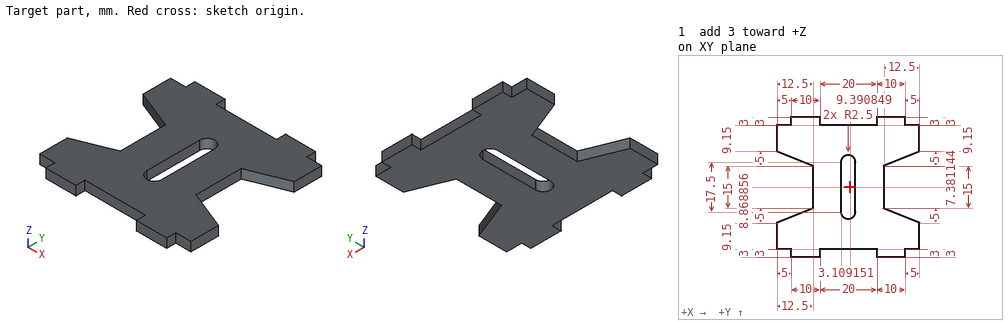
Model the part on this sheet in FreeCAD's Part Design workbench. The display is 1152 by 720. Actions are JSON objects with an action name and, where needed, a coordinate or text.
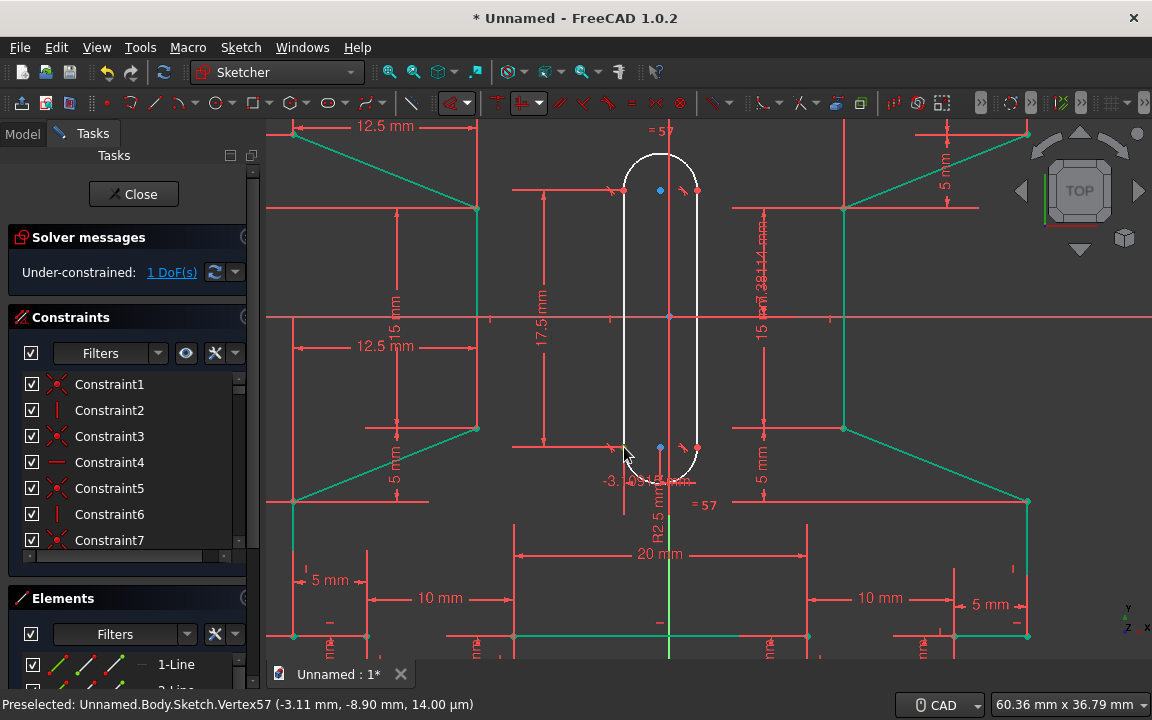
{"action": "key", "text": "i"}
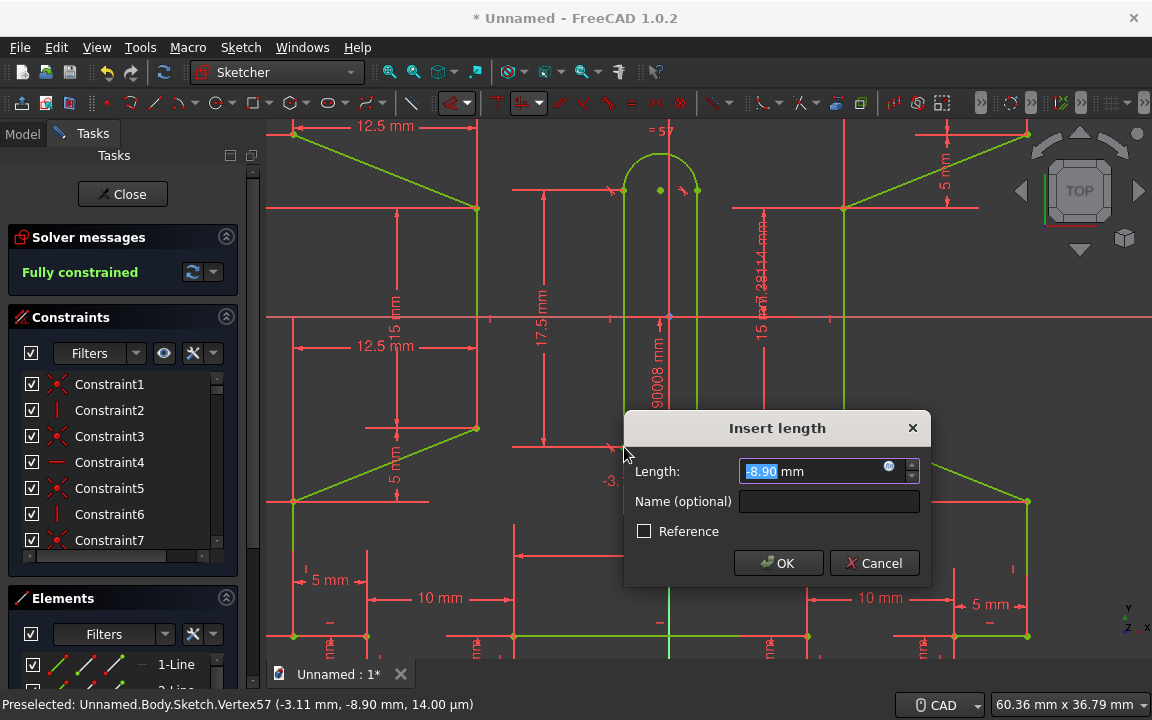
{"action": "type", "text": "-8.868856"}
{"action": "key", "text": "Return"}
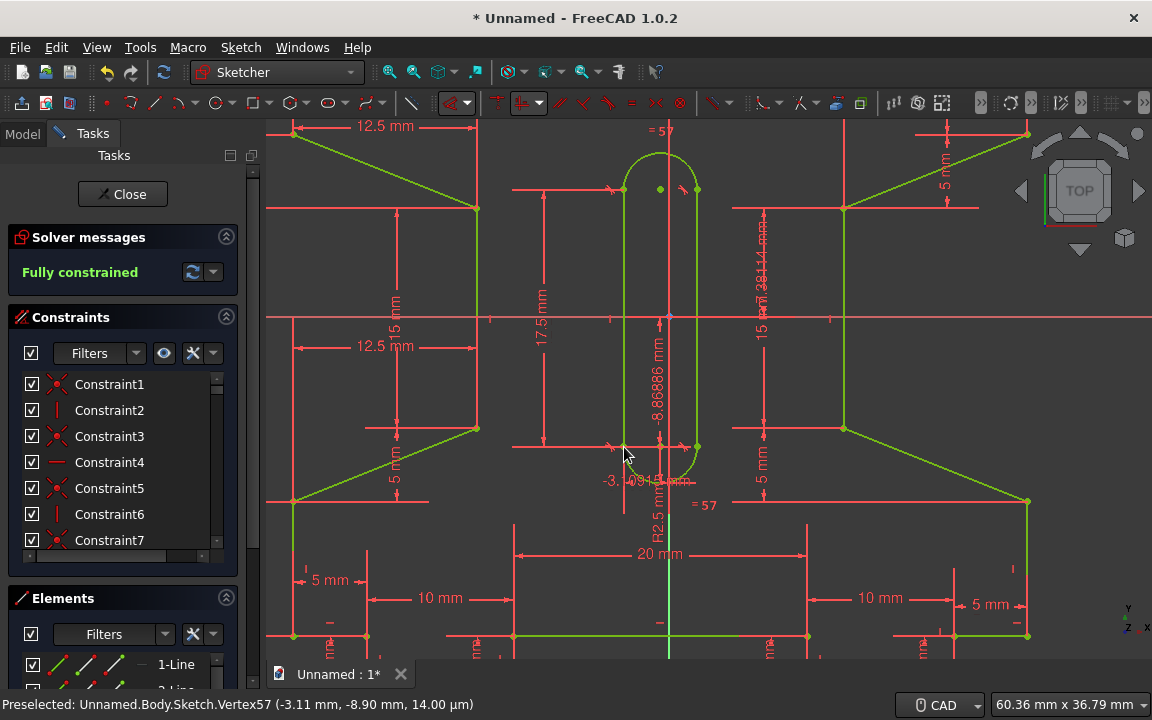
{"action": "left_click", "coordinate": [123, 194]}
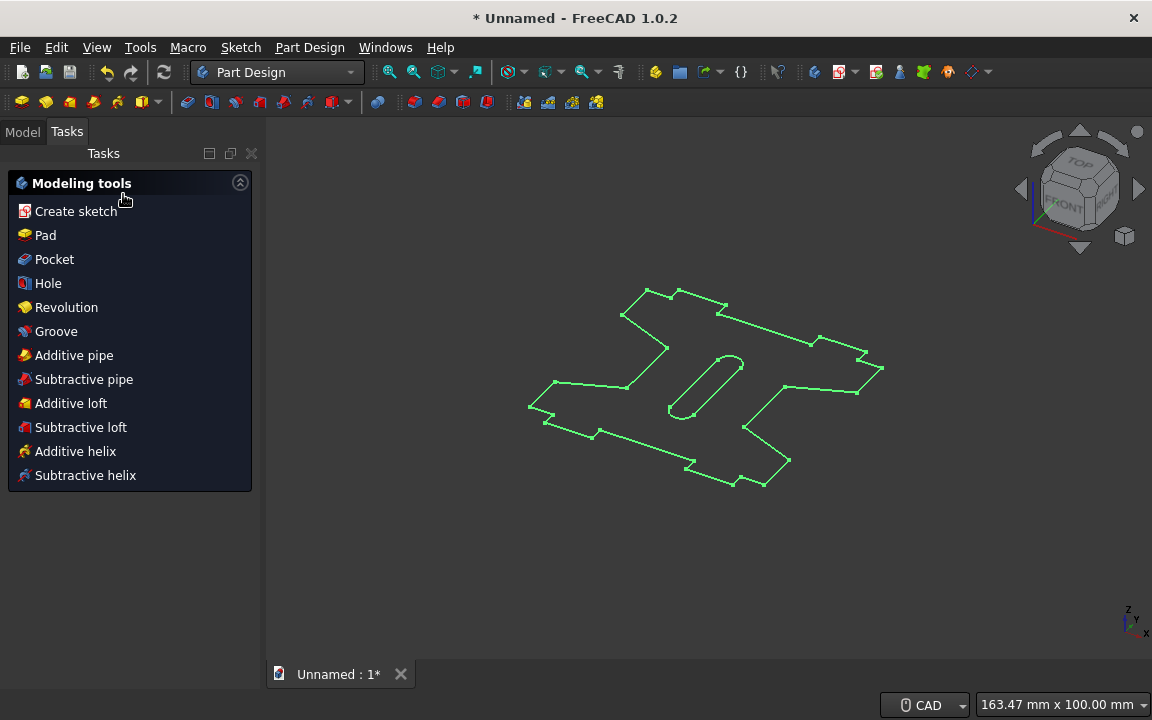
{"action": "left_click", "coordinate": [22, 102]}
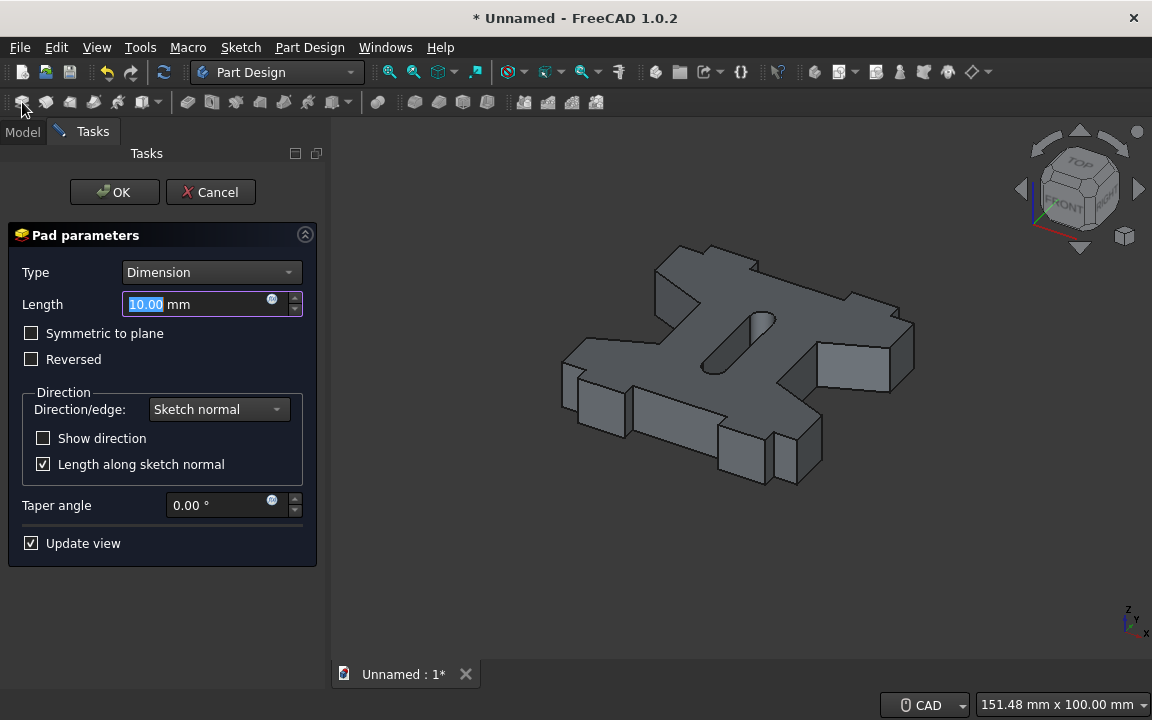
{"action": "type", "text": "3"}
{"action": "key", "text": "Tab"}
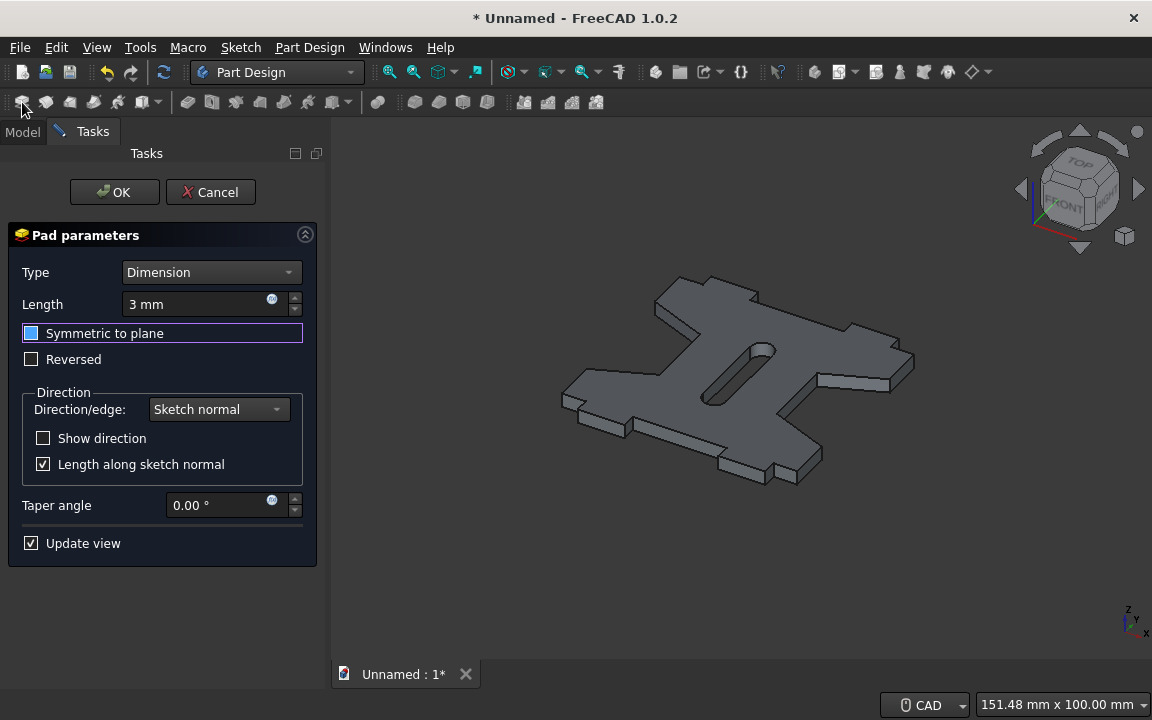
{"action": "left_click", "coordinate": [115, 192]}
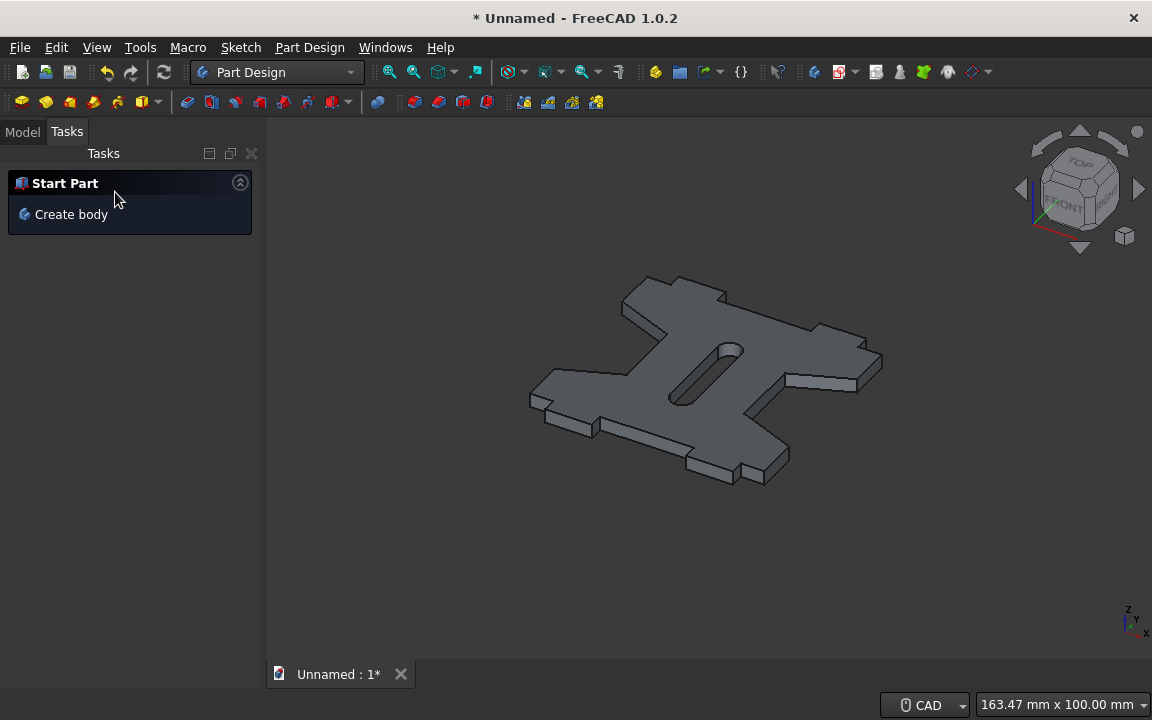
{"action": "key", "text": "0"}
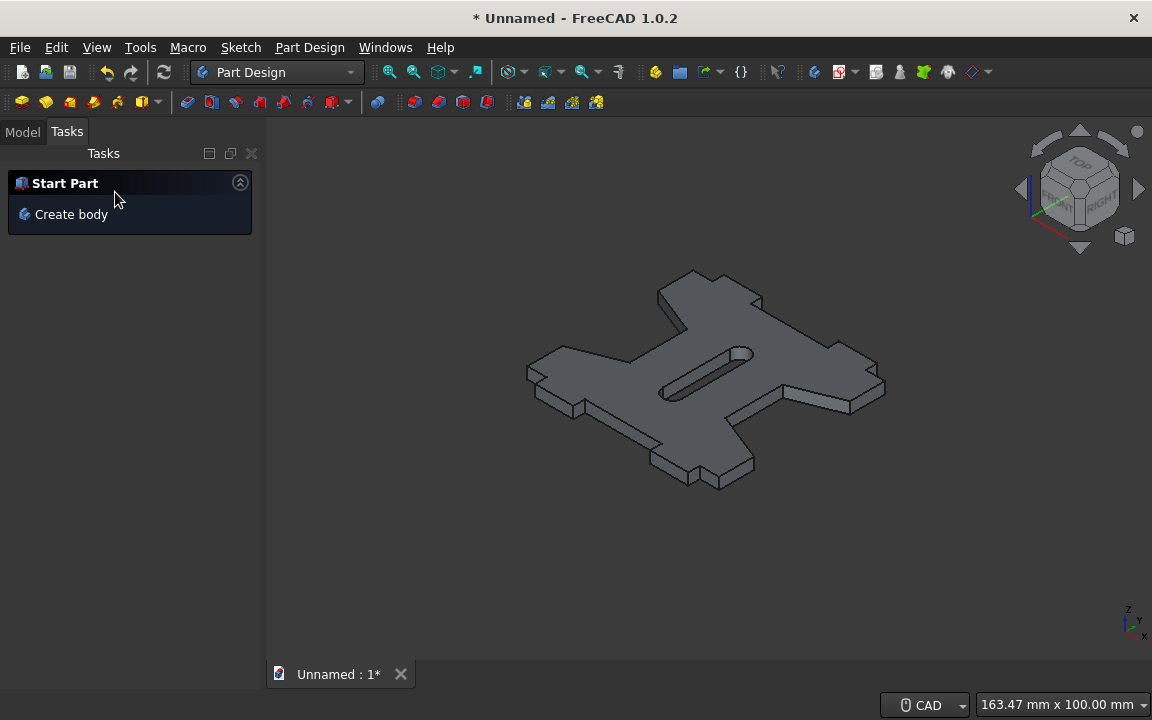
{"action": "left_click", "coordinate": [390, 72]}